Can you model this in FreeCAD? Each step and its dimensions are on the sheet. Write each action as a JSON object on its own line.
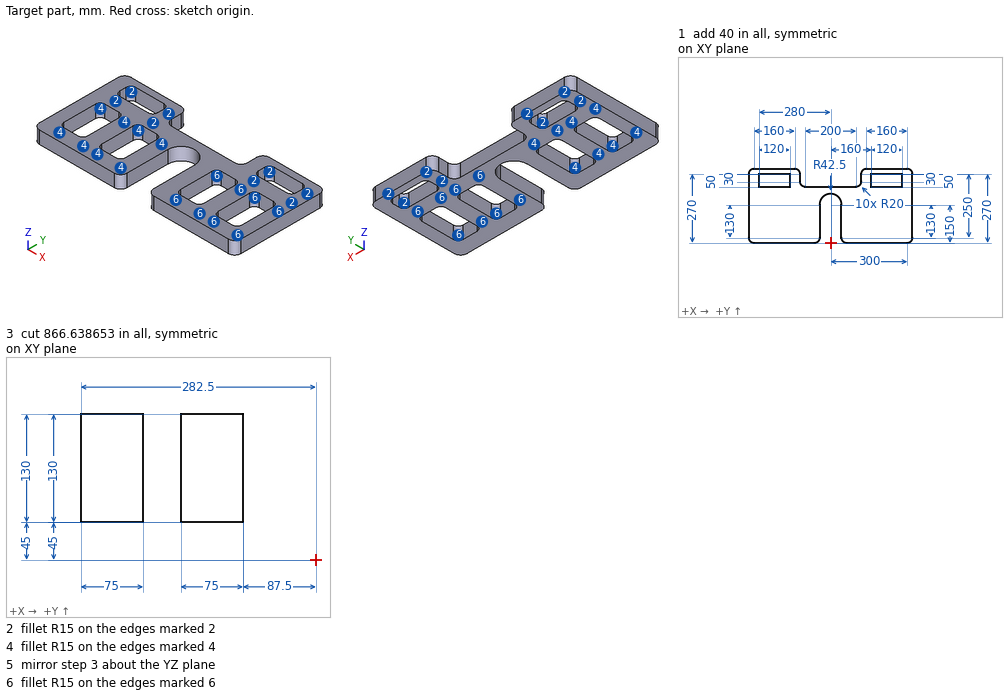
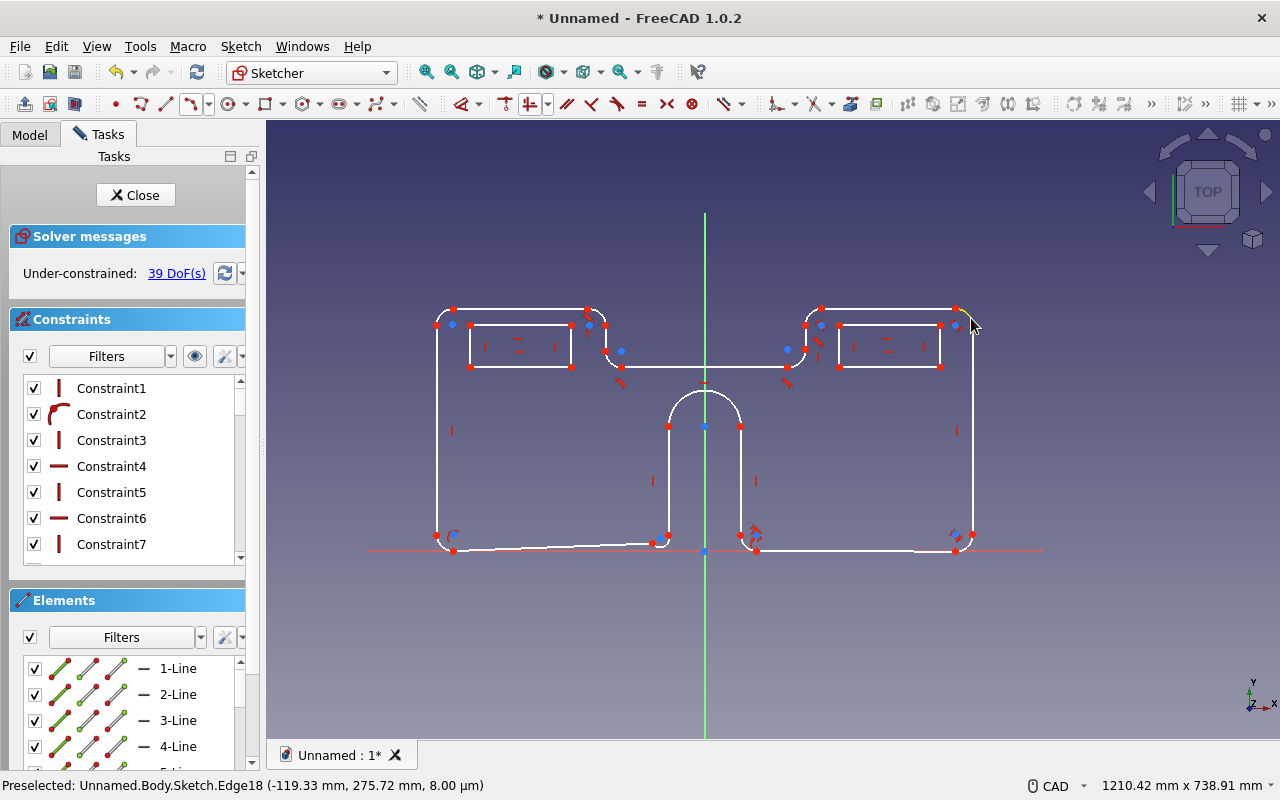
{"action": "left_click", "coordinate": [548, 309]}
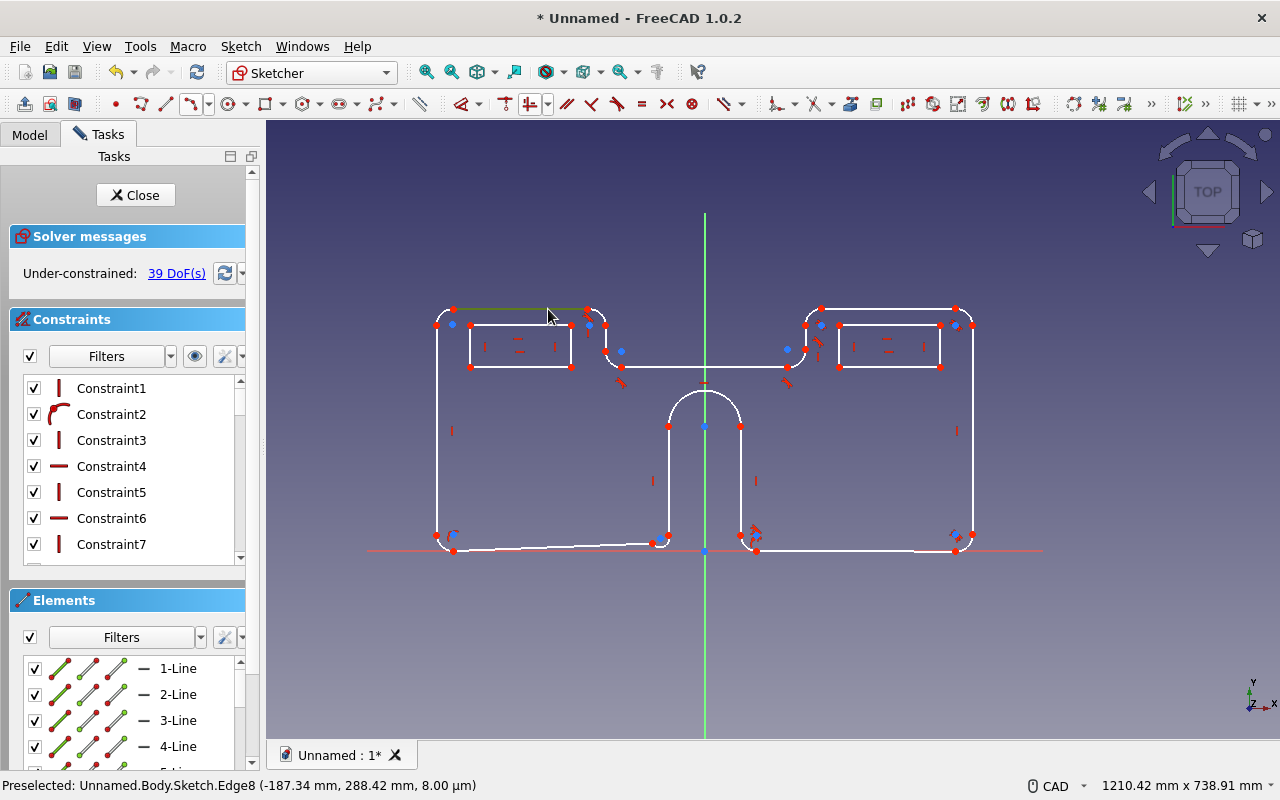
{"action": "left_click", "coordinate": [600, 313]}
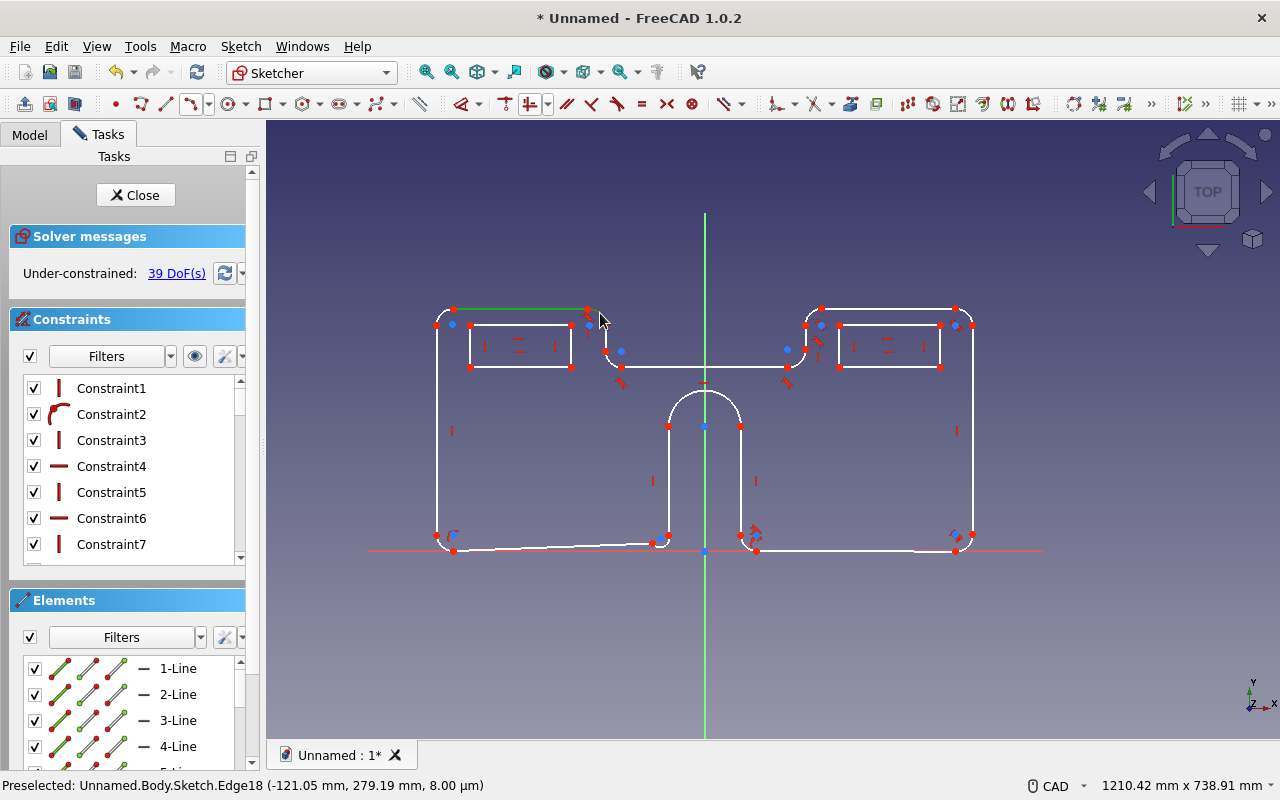
{"action": "key", "text": "t"}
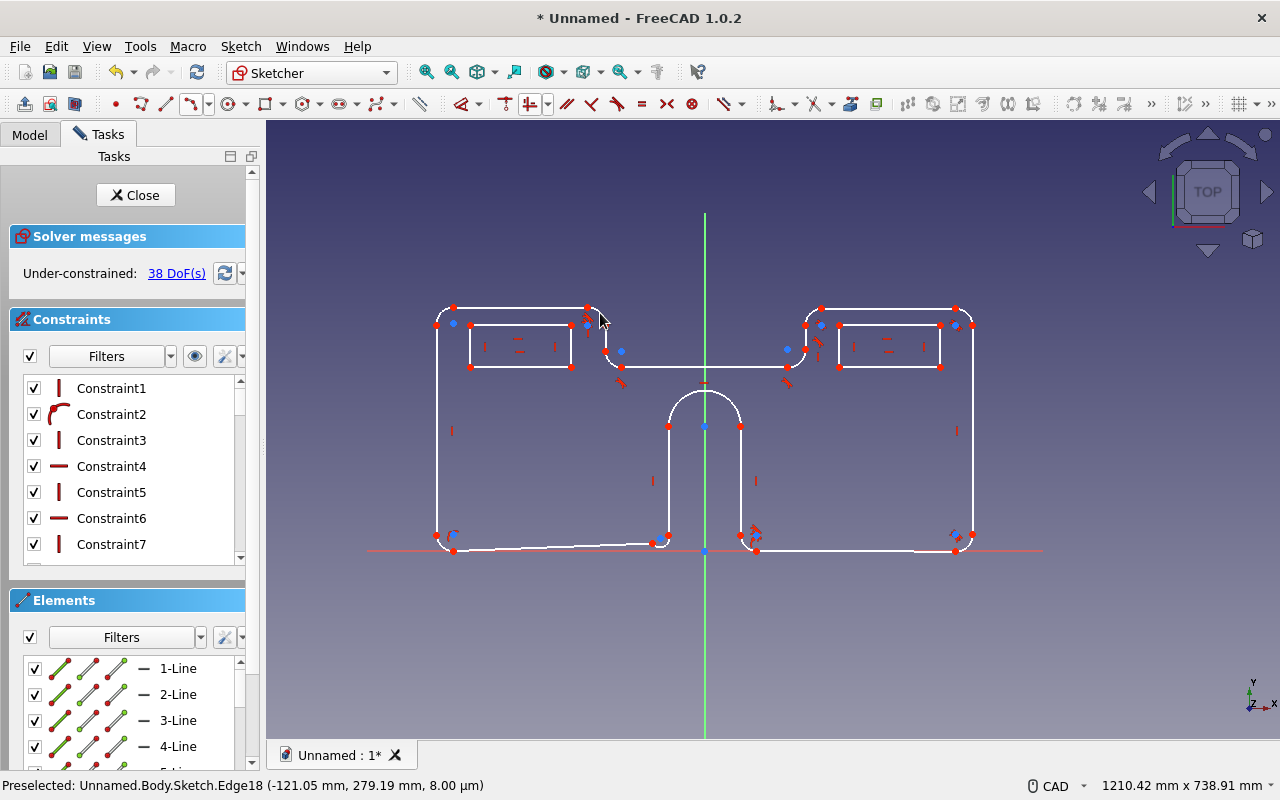
{"action": "left_click", "coordinate": [548, 308]}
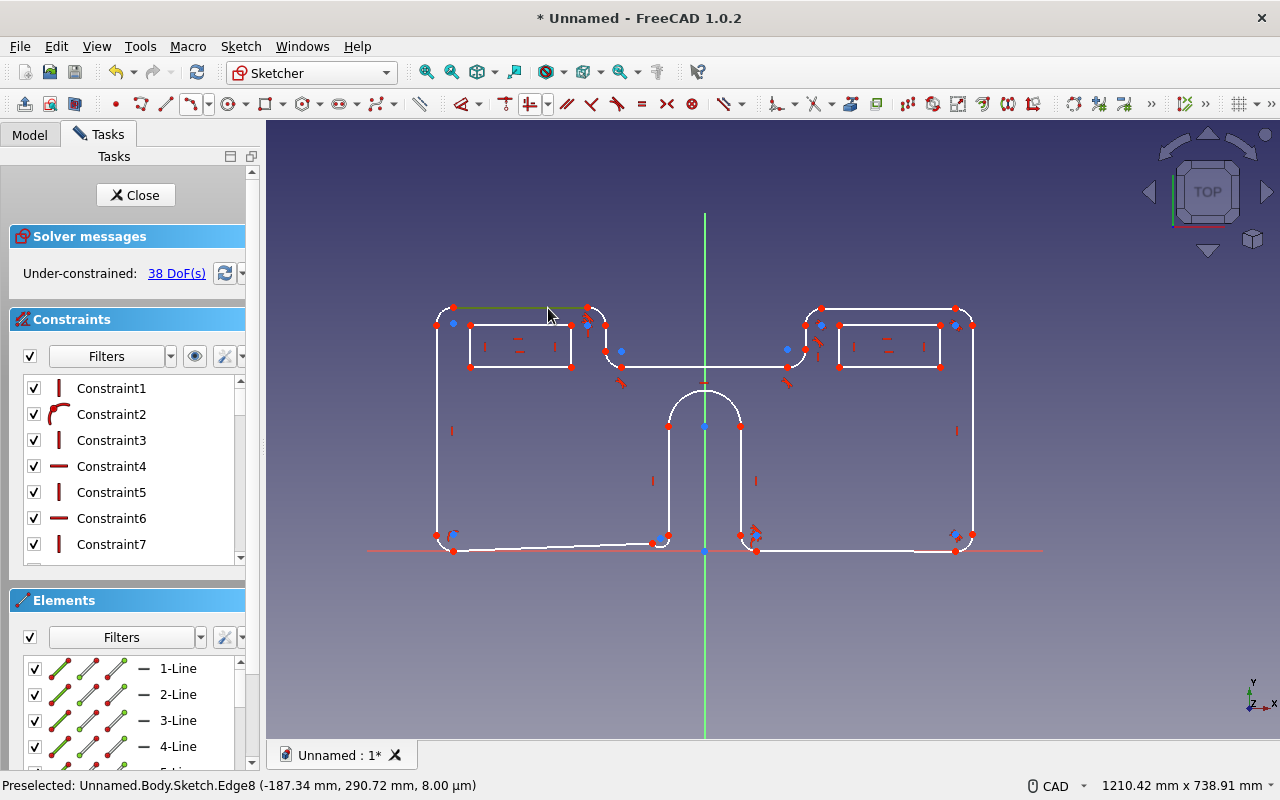
{"action": "left_click", "coordinate": [441, 313]}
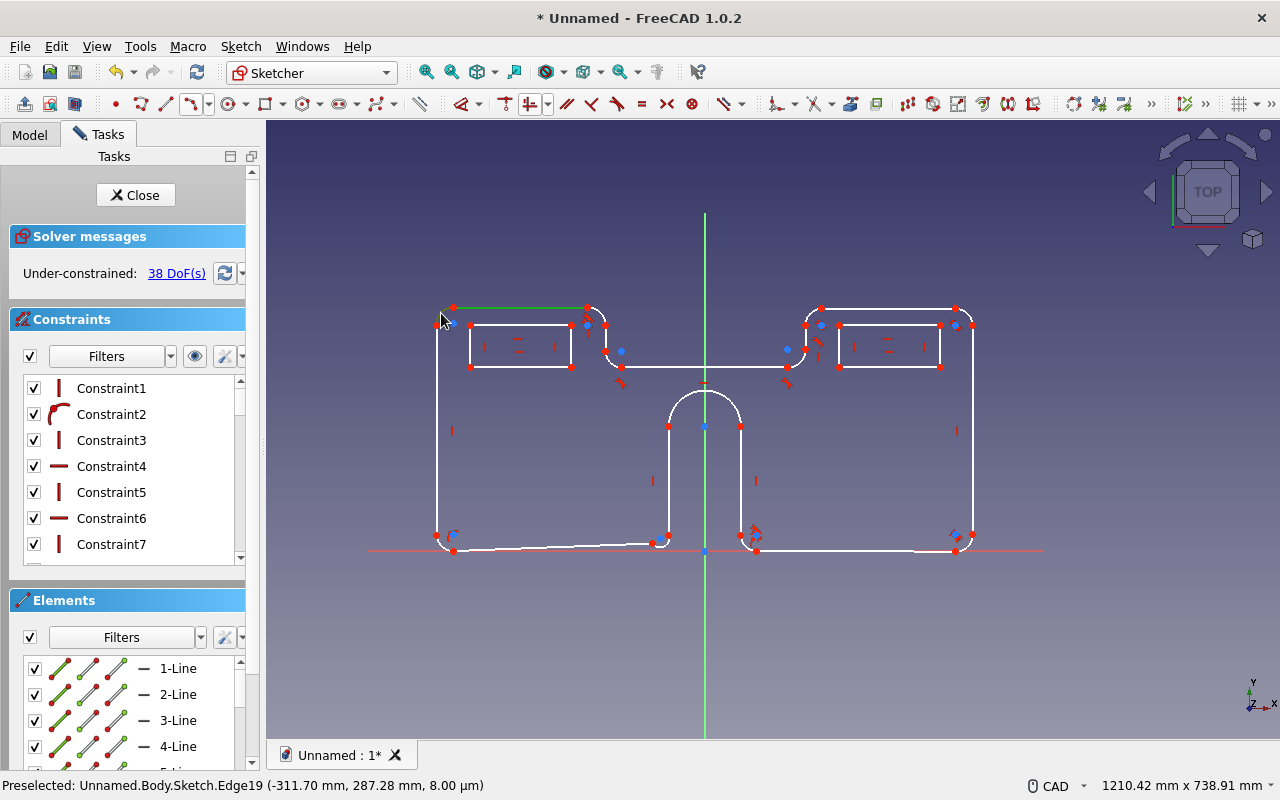
{"action": "key", "text": "t"}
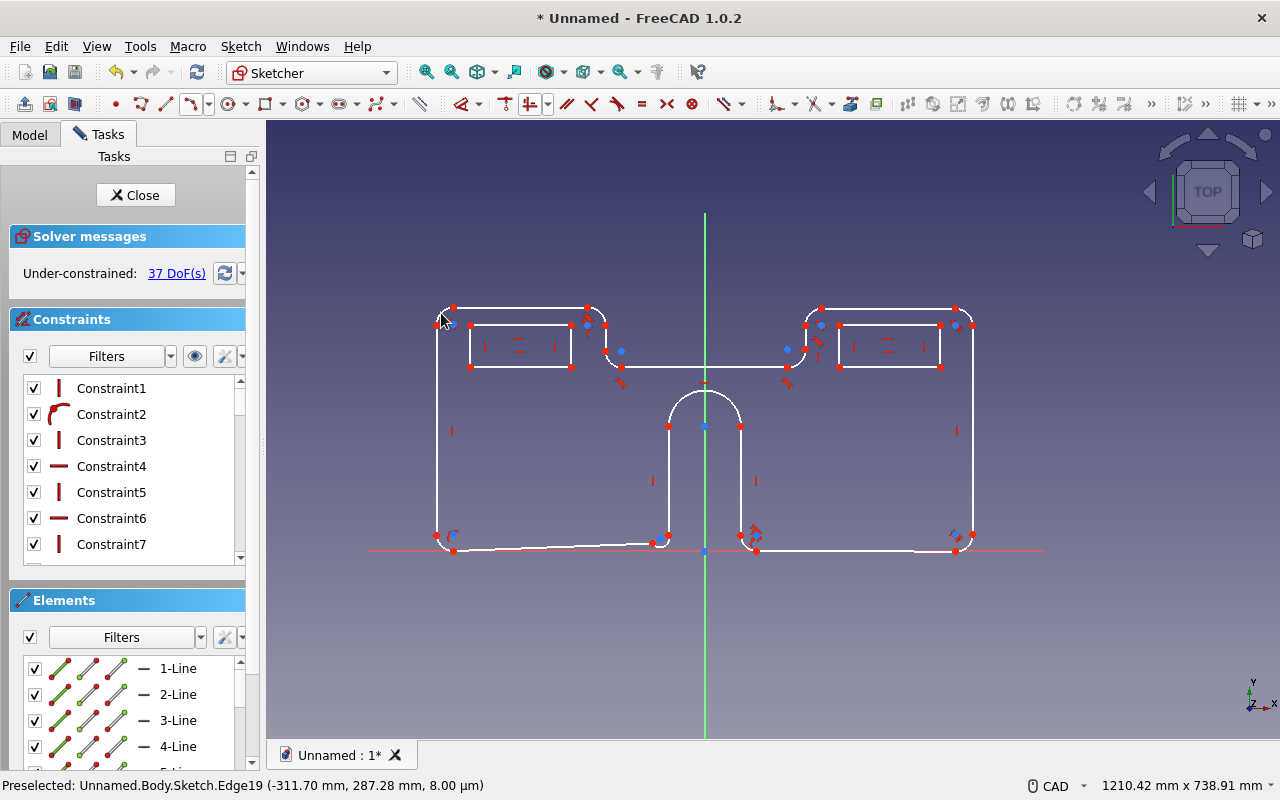
{"action": "left_click", "coordinate": [437, 388]}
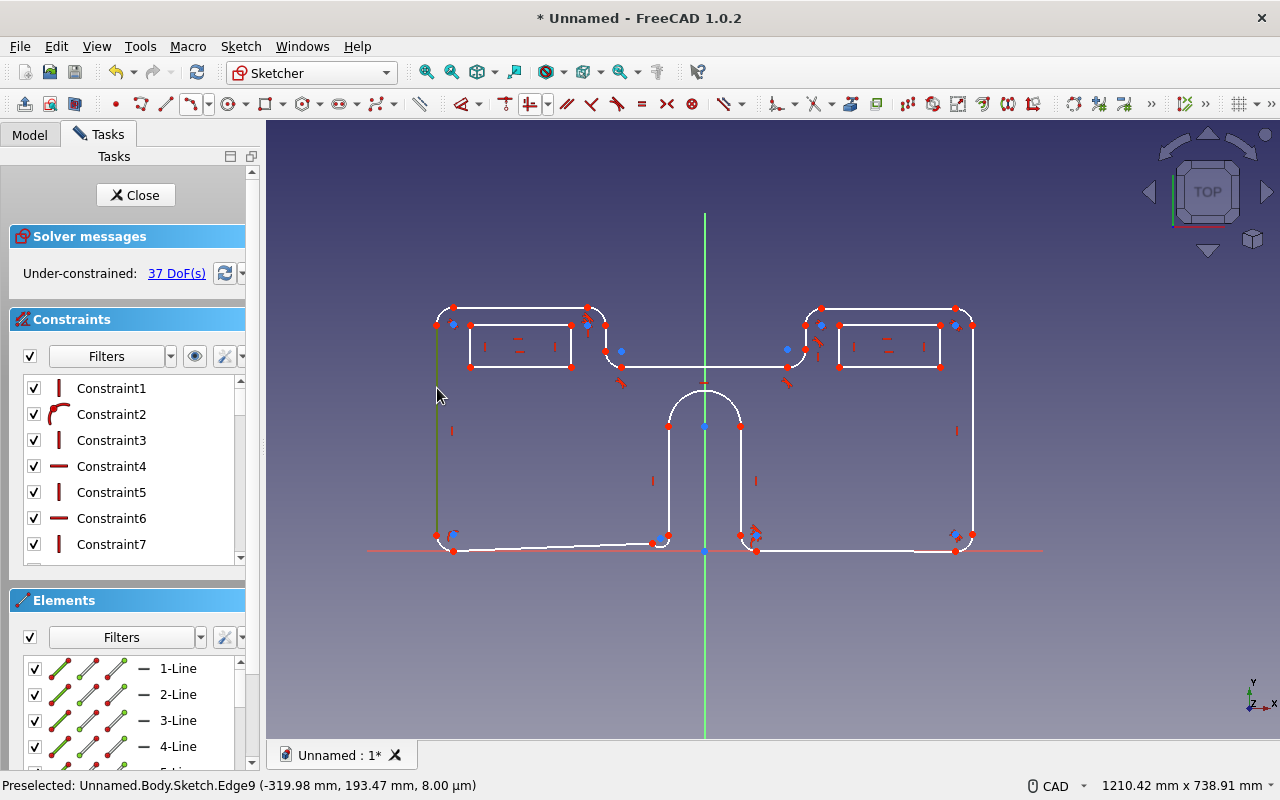
{"action": "left_click", "coordinate": [442, 313]}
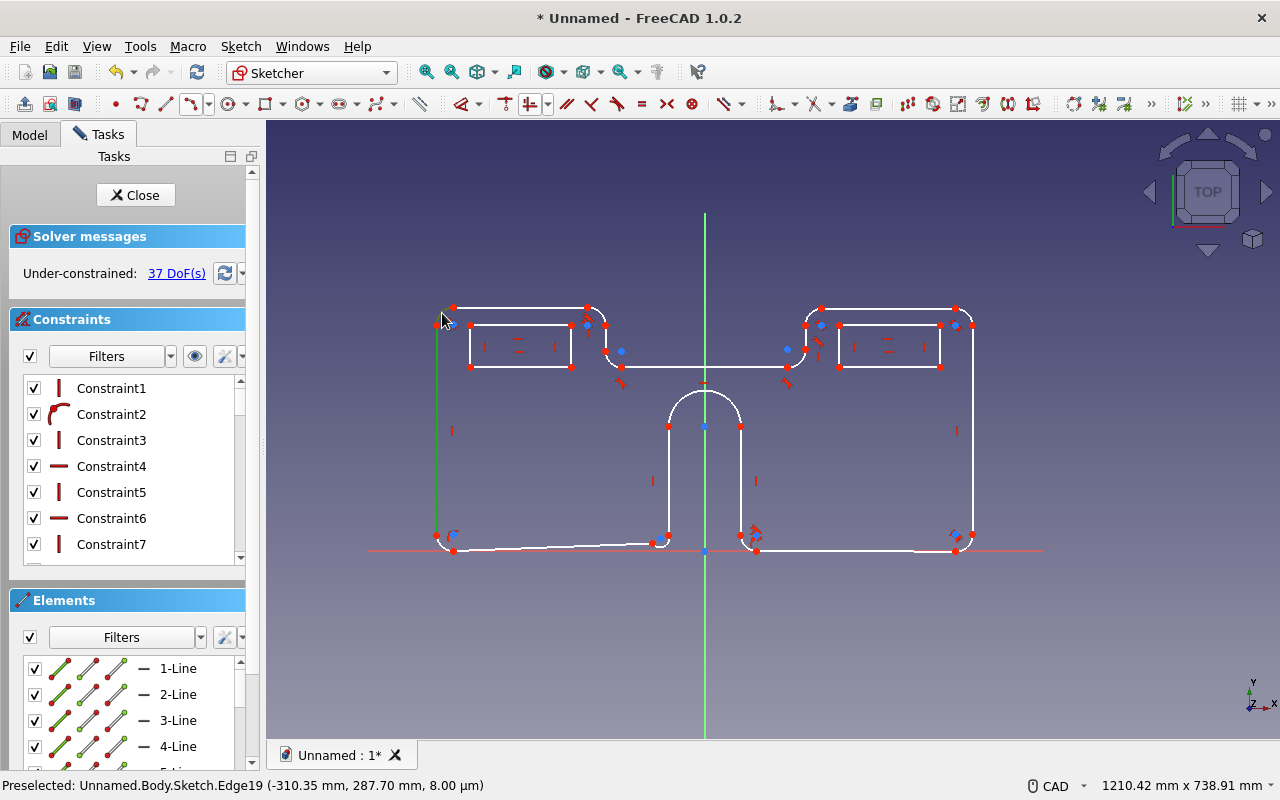
{"action": "key", "text": "t"}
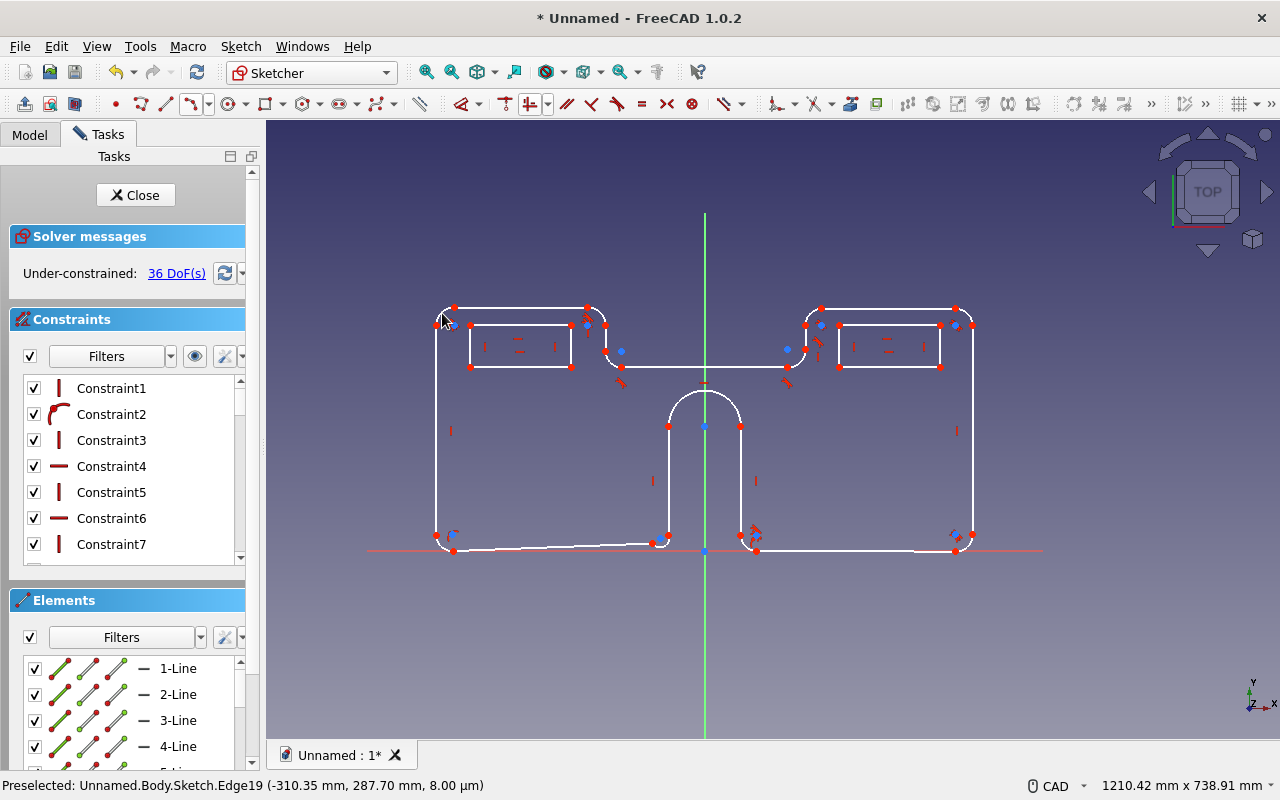
{"action": "left_click", "coordinate": [436, 388]}